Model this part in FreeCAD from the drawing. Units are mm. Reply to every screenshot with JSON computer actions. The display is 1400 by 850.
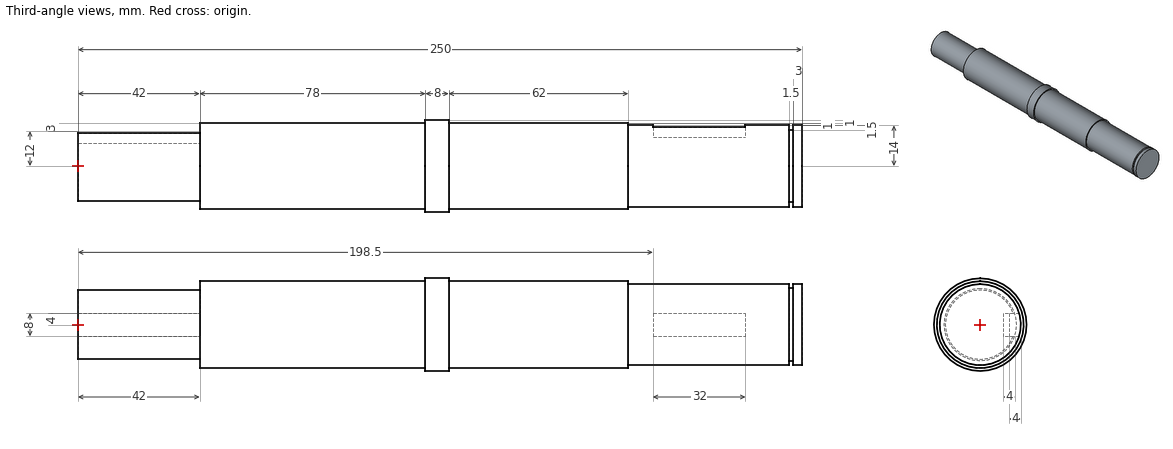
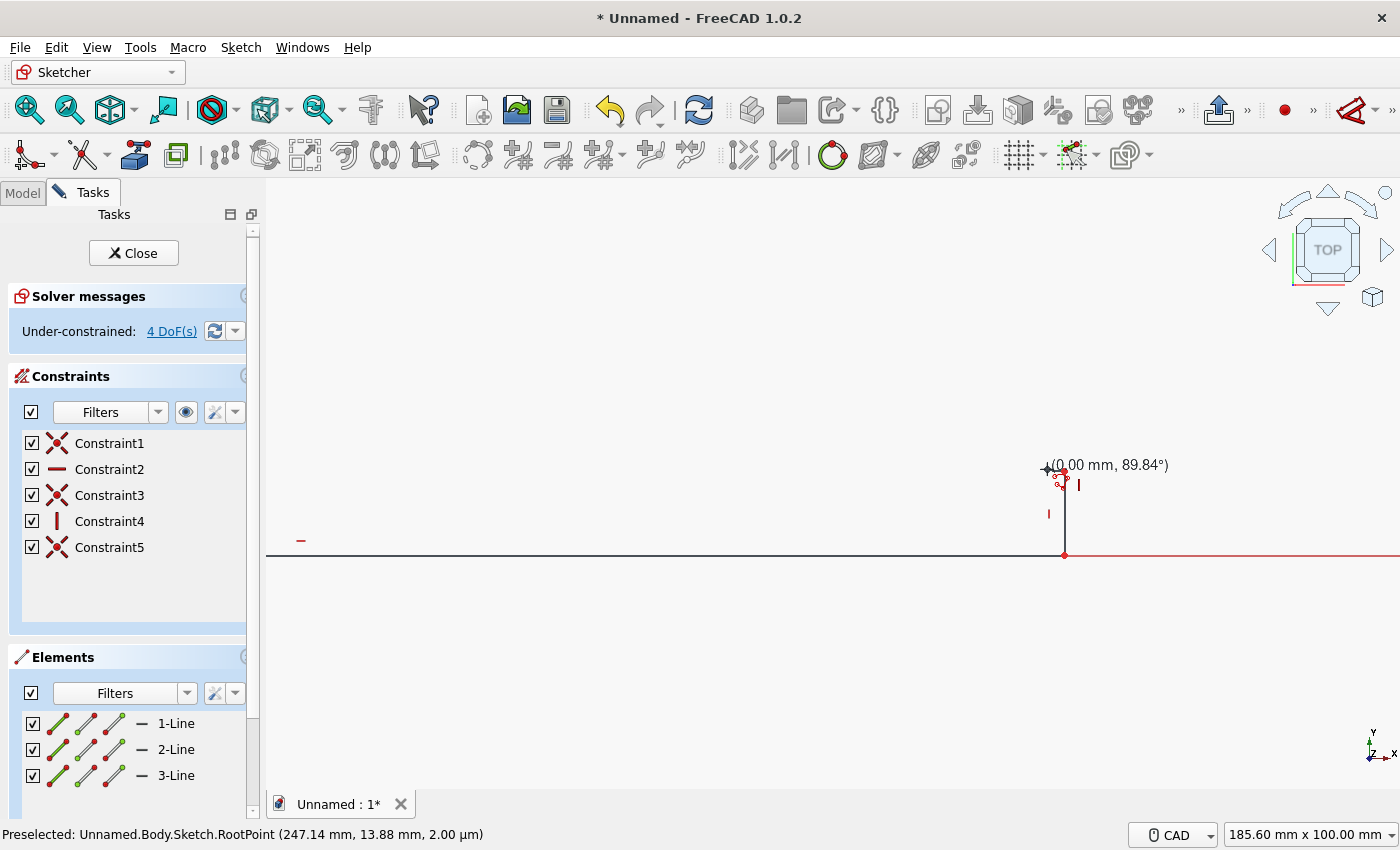
{"action": "scroll", "coordinate": [1047, 479], "scroll_direction": "up", "scroll_amount": 3}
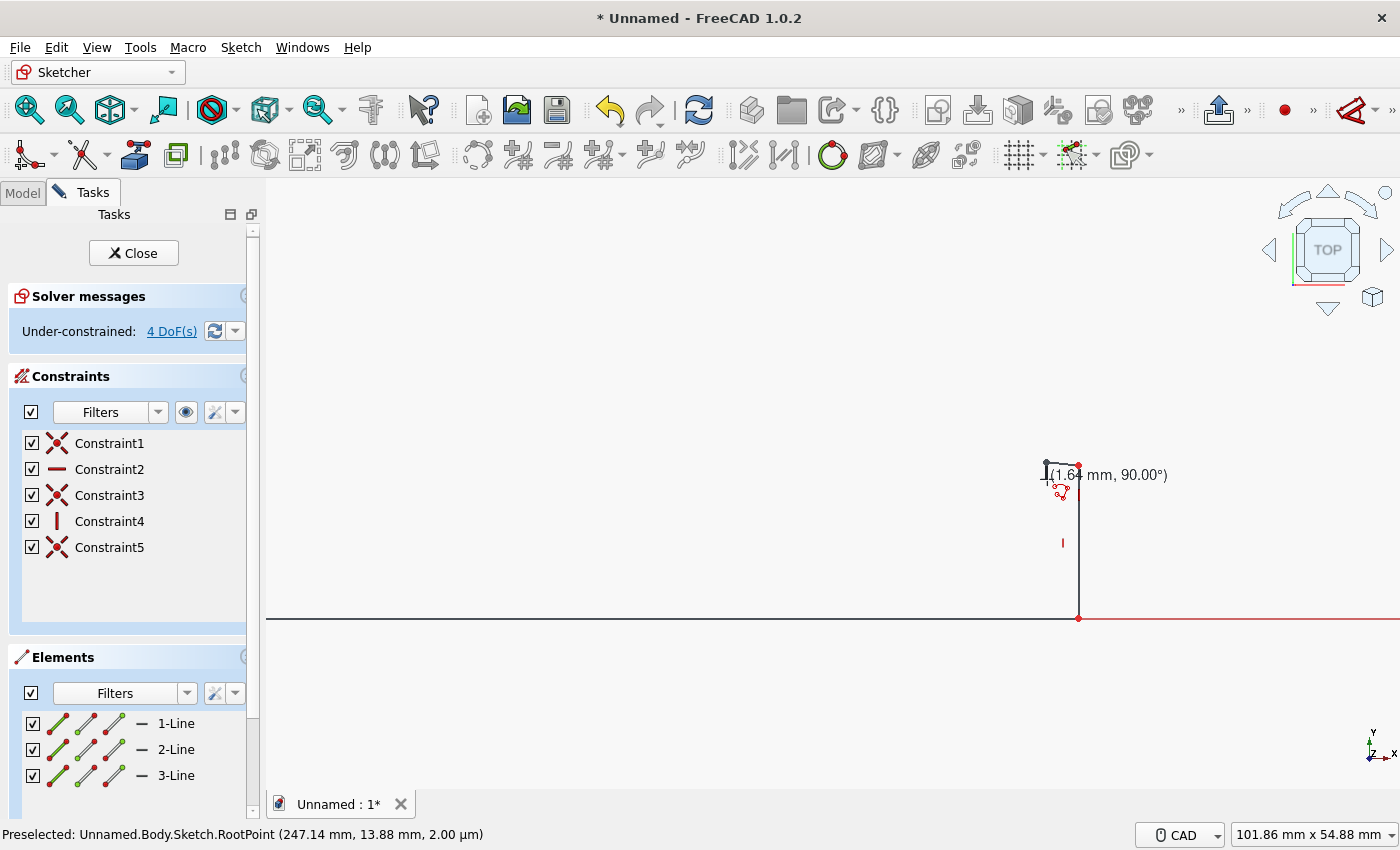
{"action": "left_click", "coordinate": [1046, 479]}
{"action": "left_click", "coordinate": [1030, 479]}
{"action": "left_click", "coordinate": [1030, 463]}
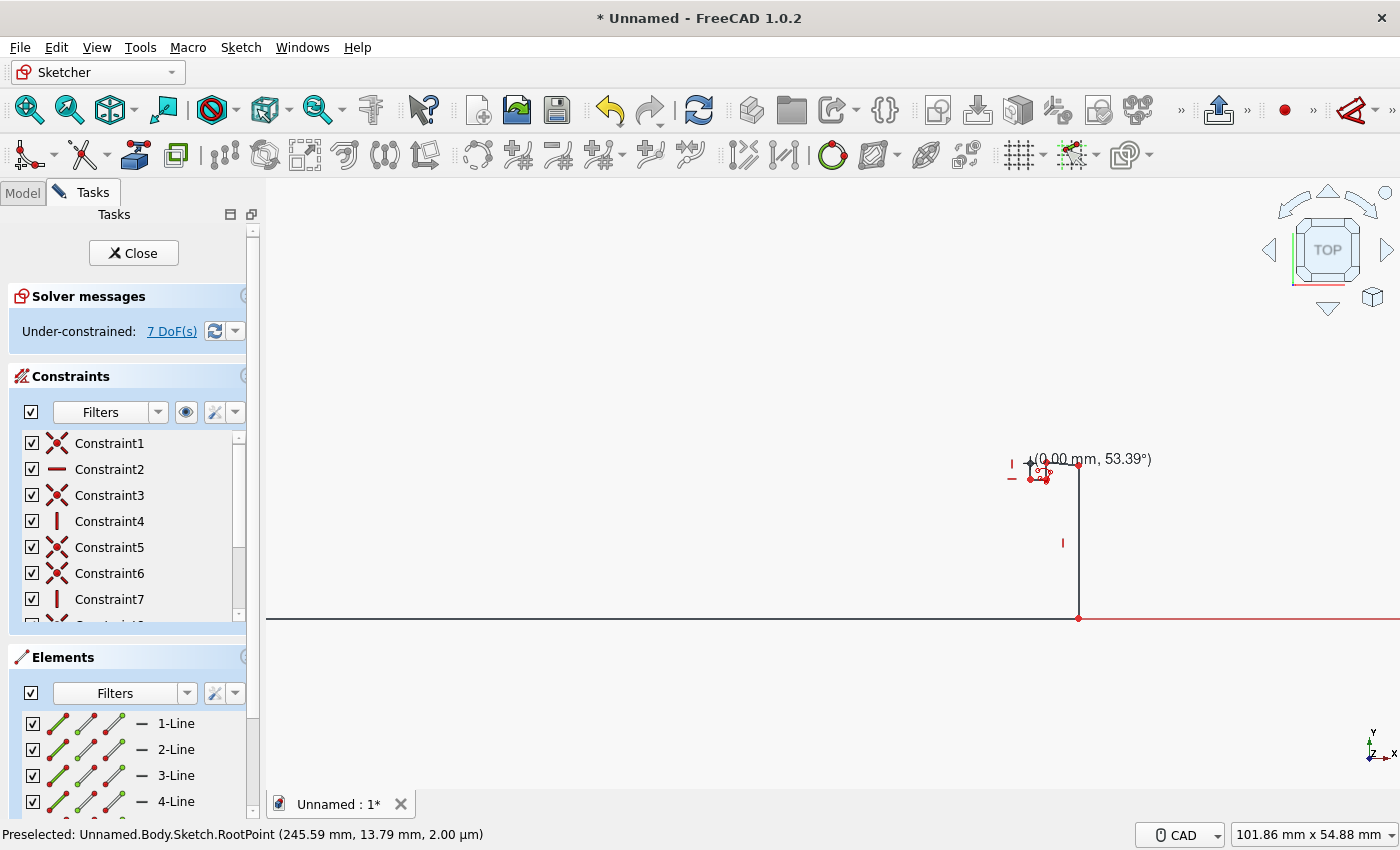
{"action": "scroll", "coordinate": [1117, 468], "scroll_direction": "down", "scroll_amount": 7}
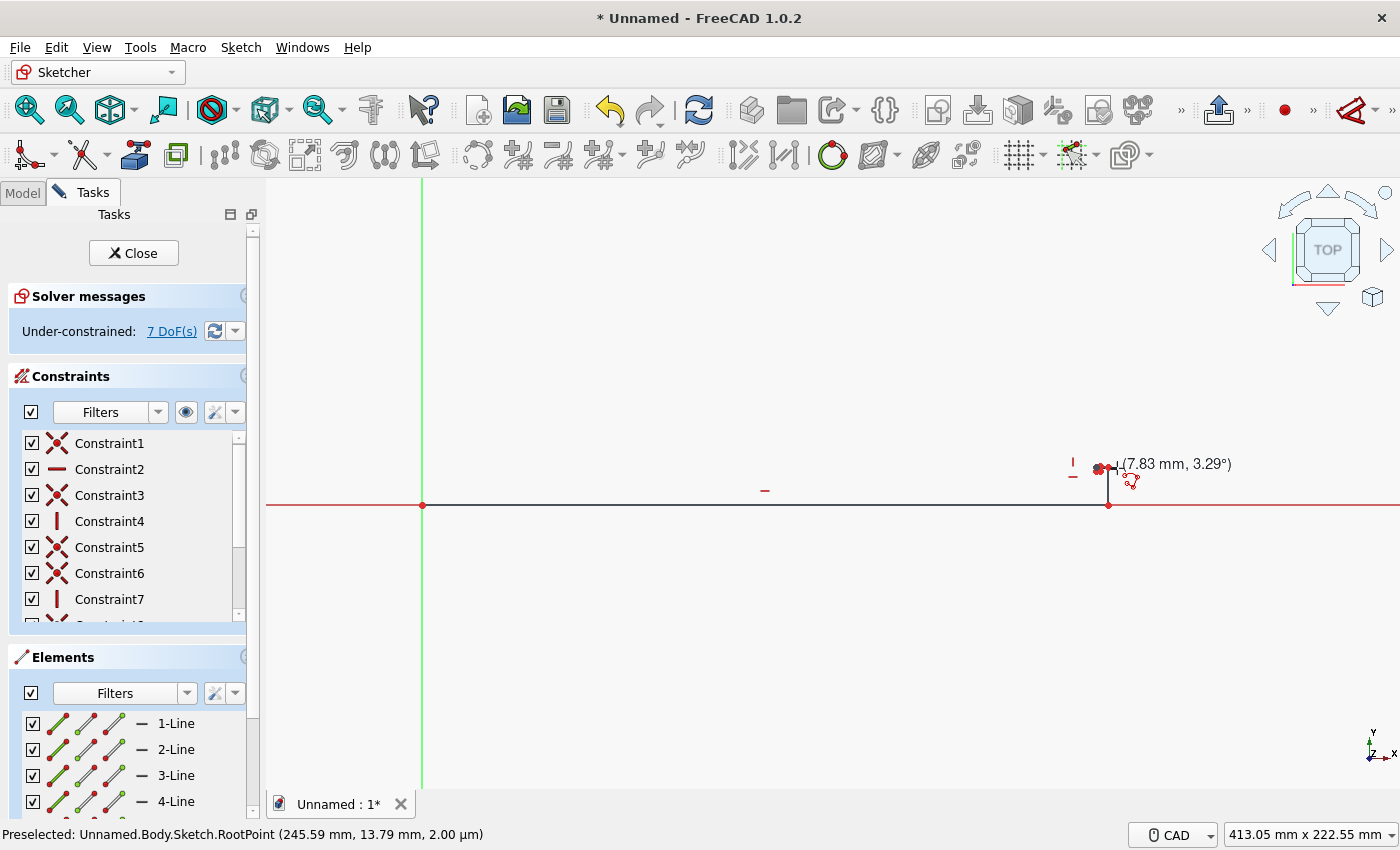
{"action": "left_click", "coordinate": [944, 467]}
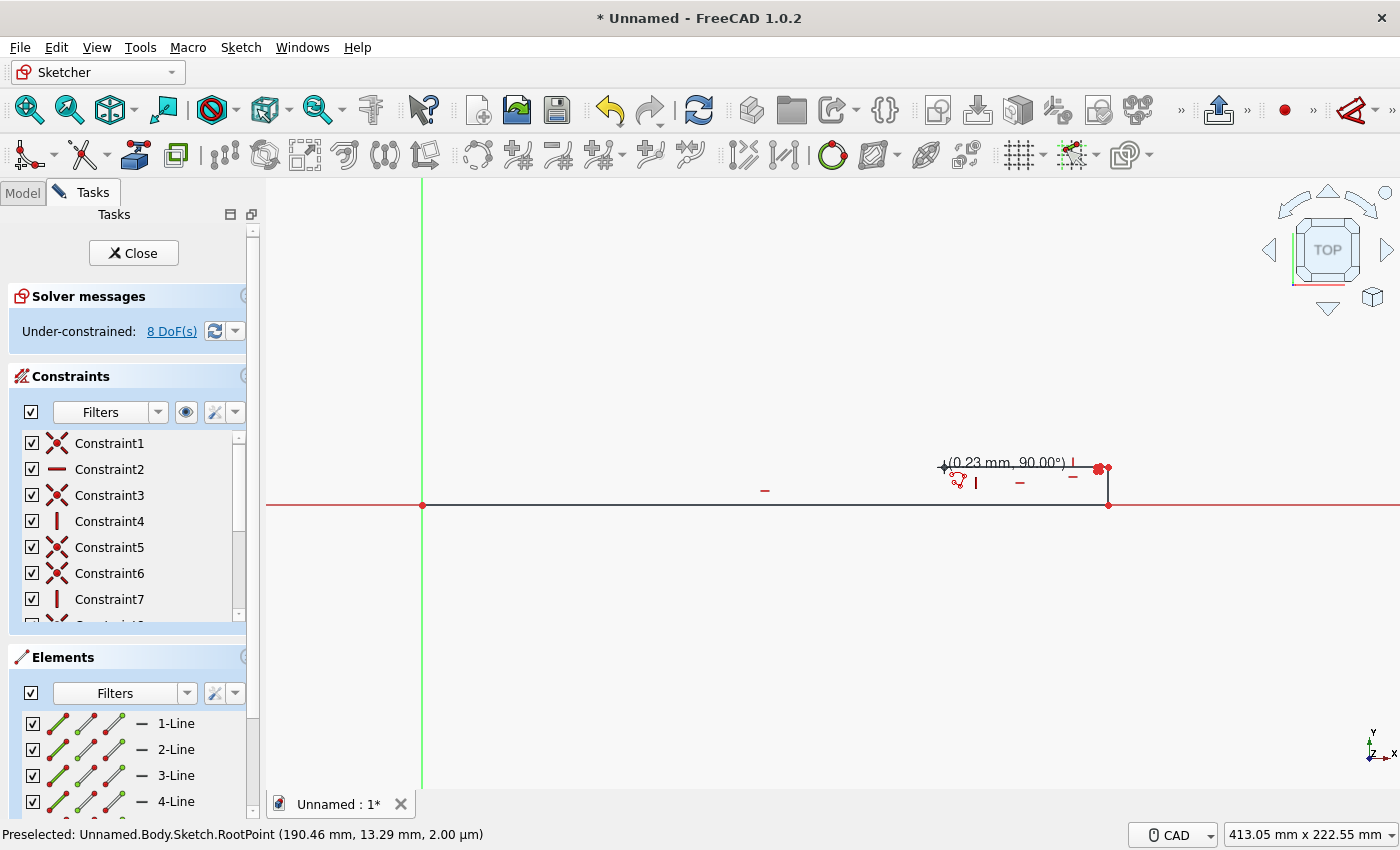
{"action": "scroll", "coordinate": [944, 464], "scroll_direction": "up", "scroll_amount": 9}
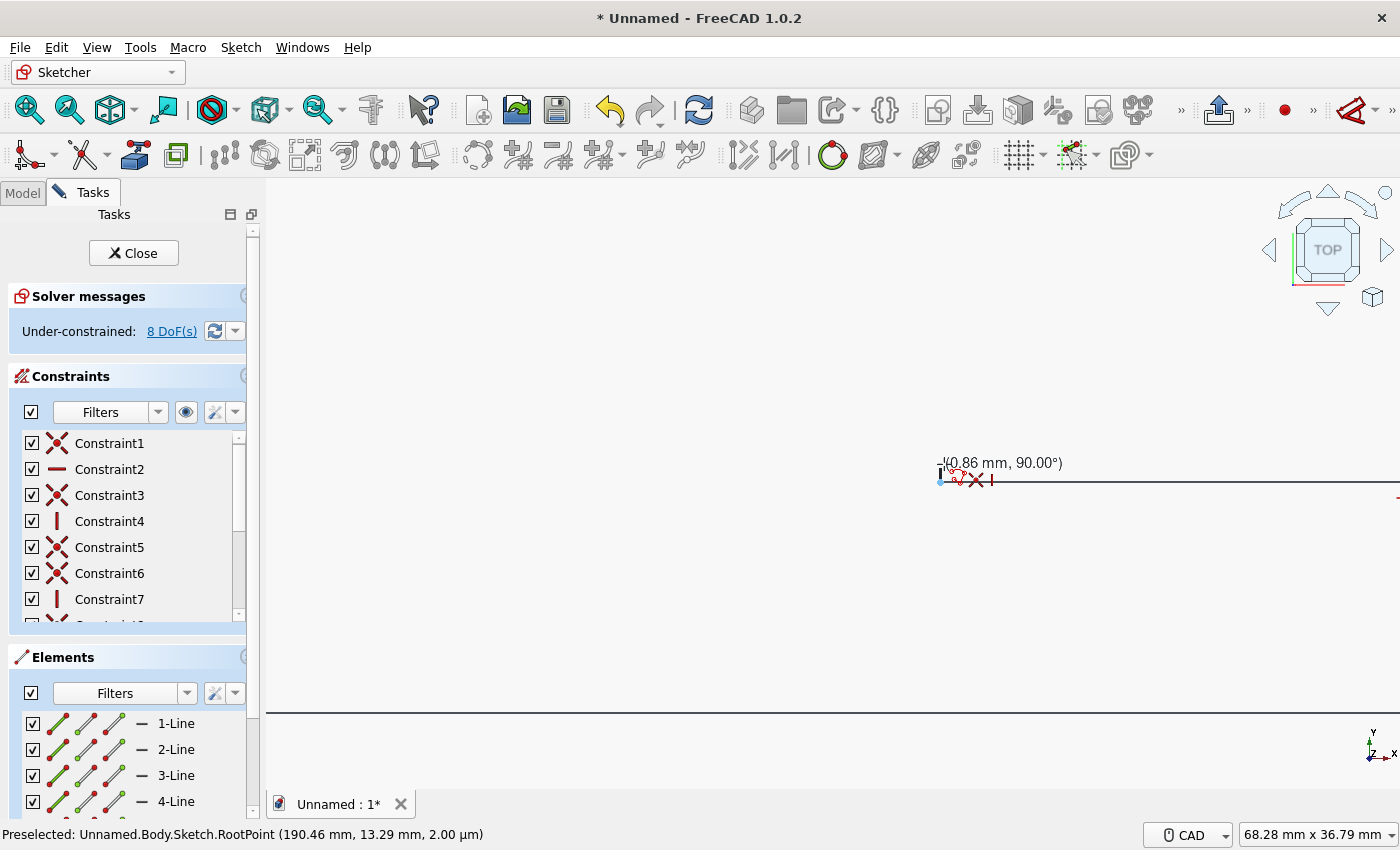
{"action": "left_click", "coordinate": [941, 463]}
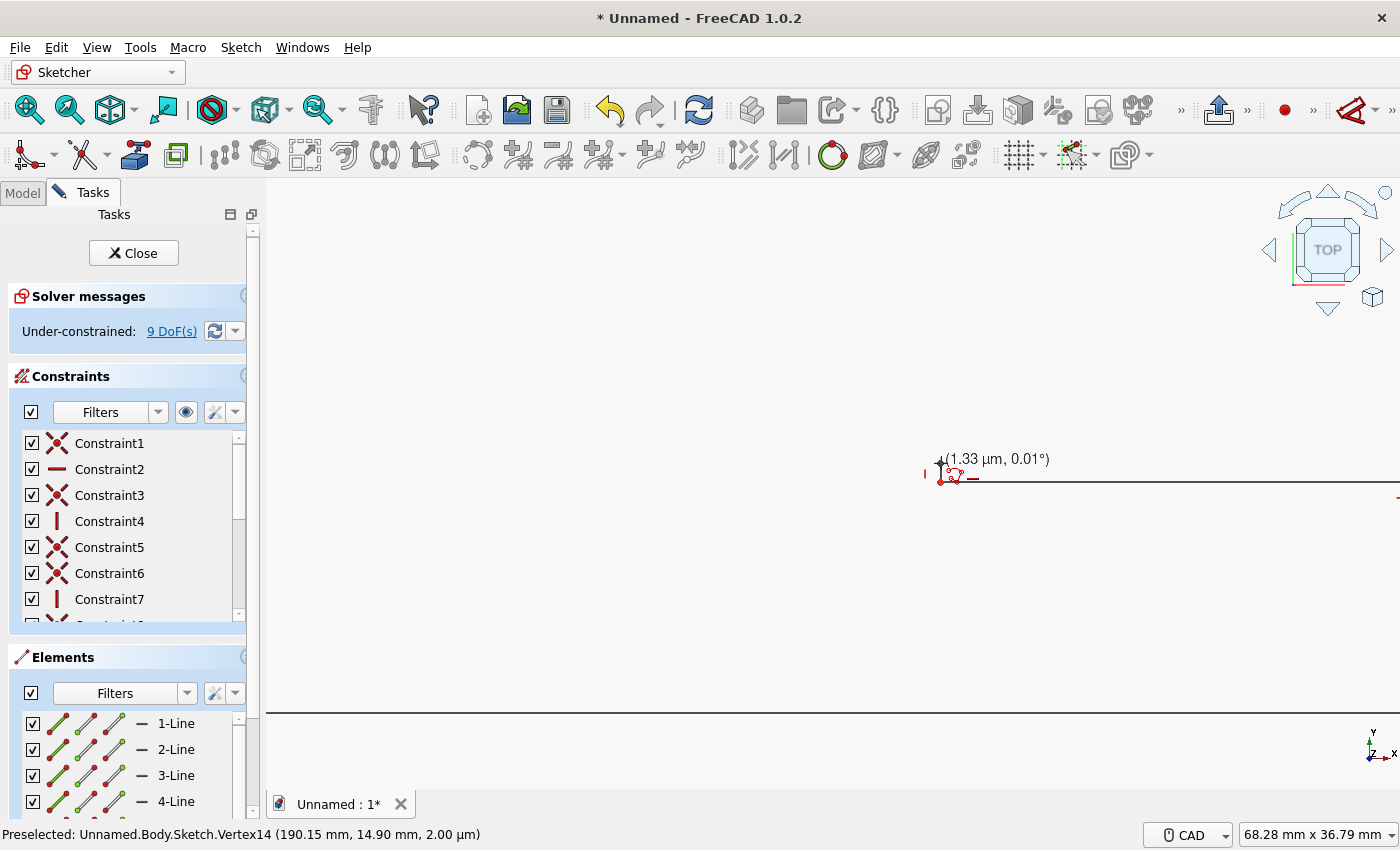
{"action": "scroll", "coordinate": [944, 464], "scroll_direction": "down", "scroll_amount": 9}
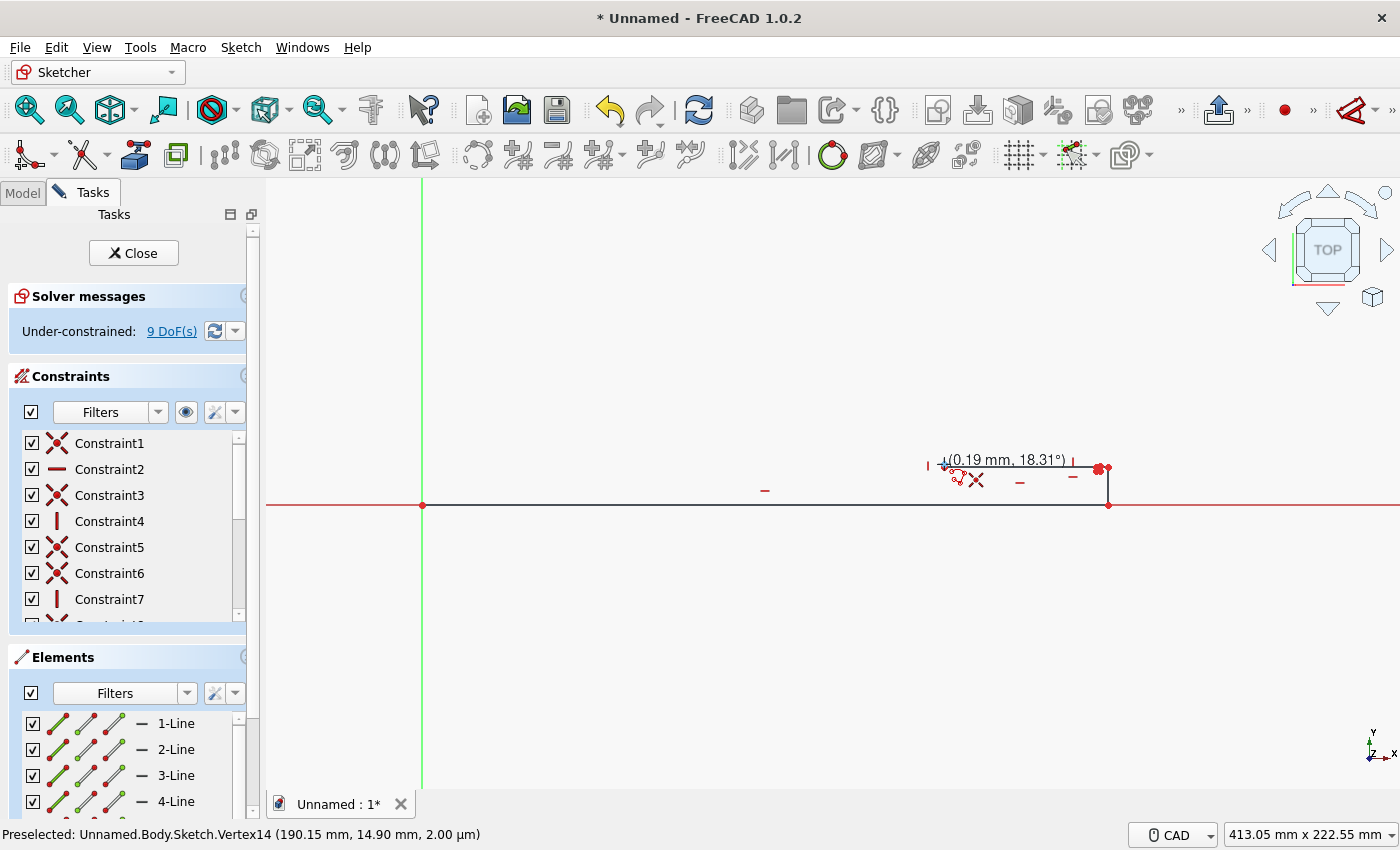
{"action": "left_click", "coordinate": [774, 464]}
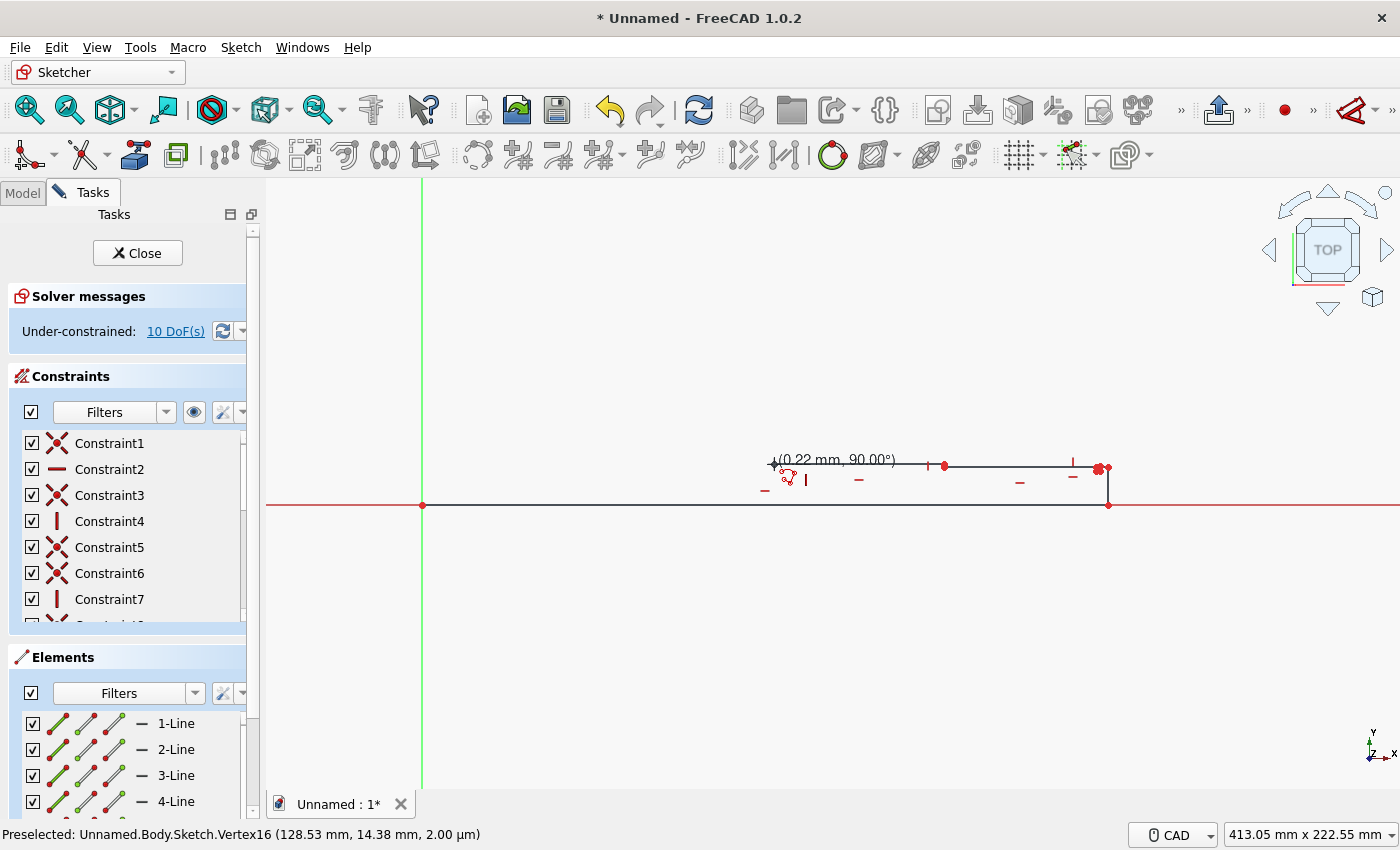
{"action": "scroll", "coordinate": [774, 462], "scroll_direction": "up", "scroll_amount": 9}